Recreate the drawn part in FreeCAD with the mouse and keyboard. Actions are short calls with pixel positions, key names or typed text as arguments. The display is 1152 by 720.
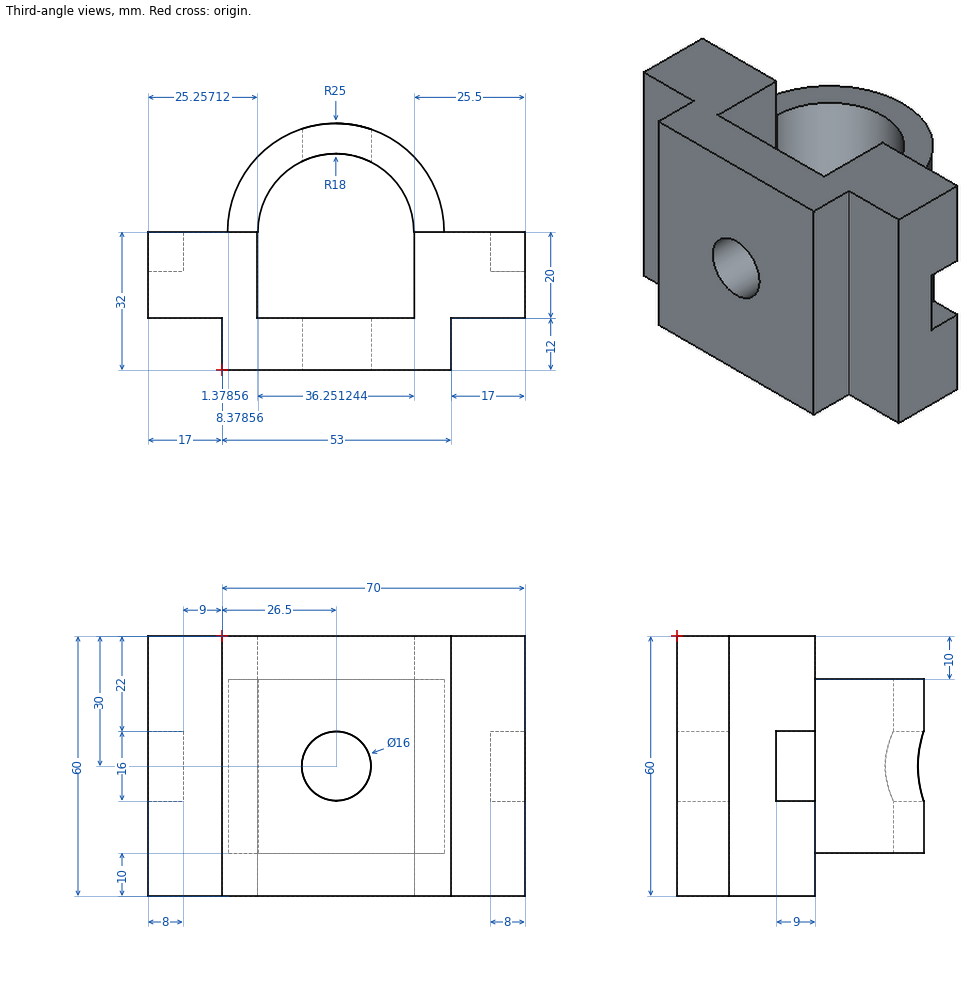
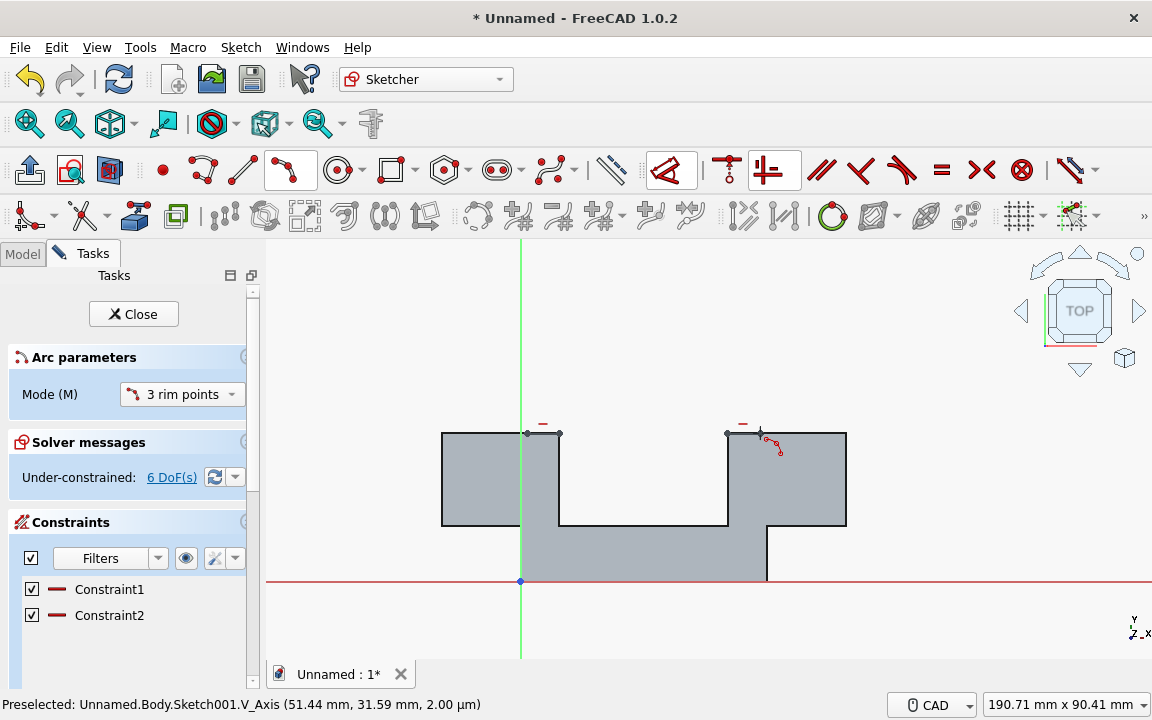
click(560, 434)
click(727, 434)
click(644, 349)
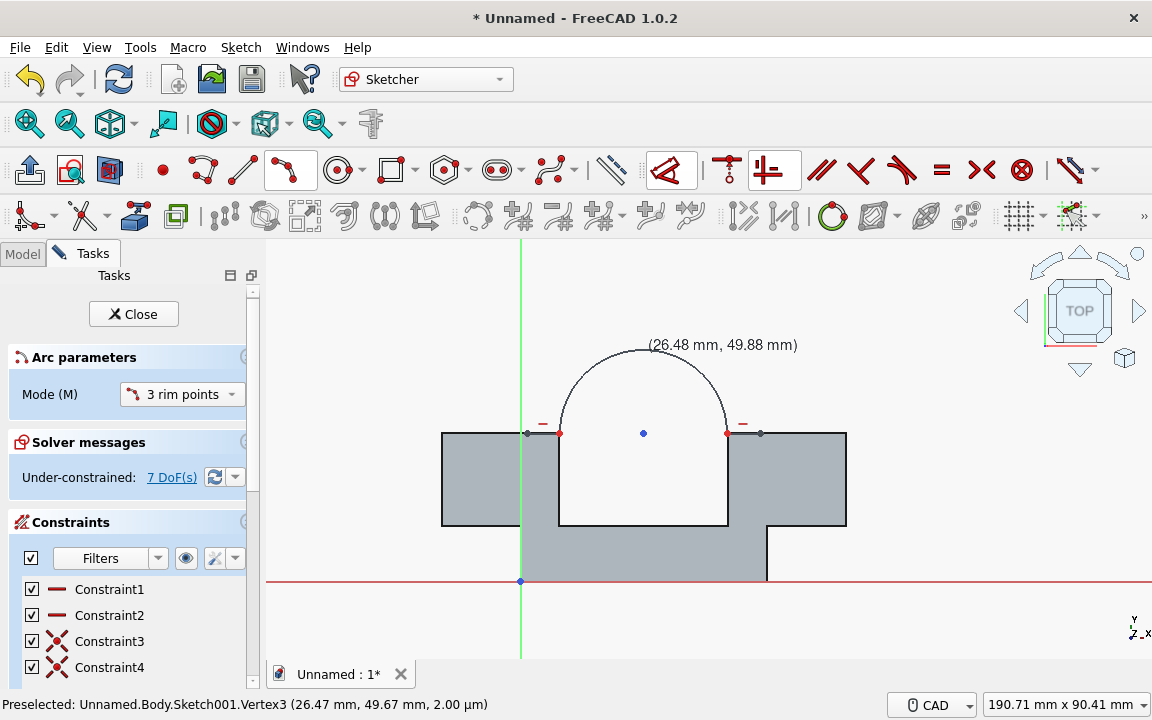
click(760, 434)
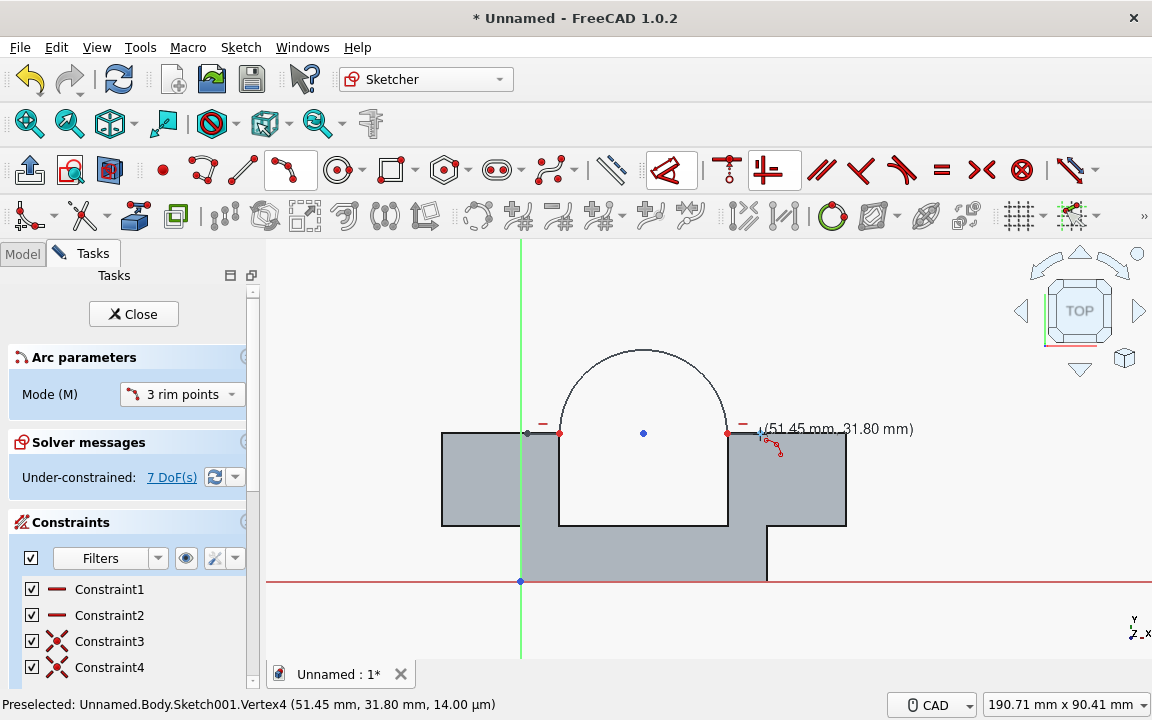
scroll(527, 433, up, 5)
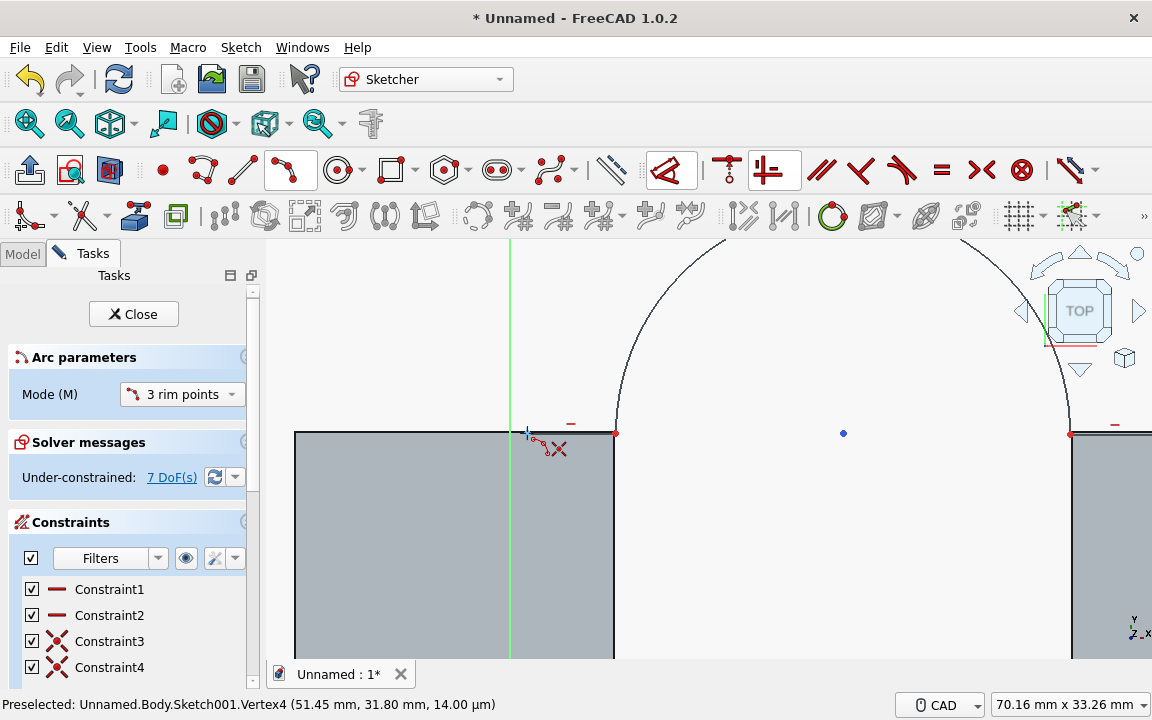
click(528, 434)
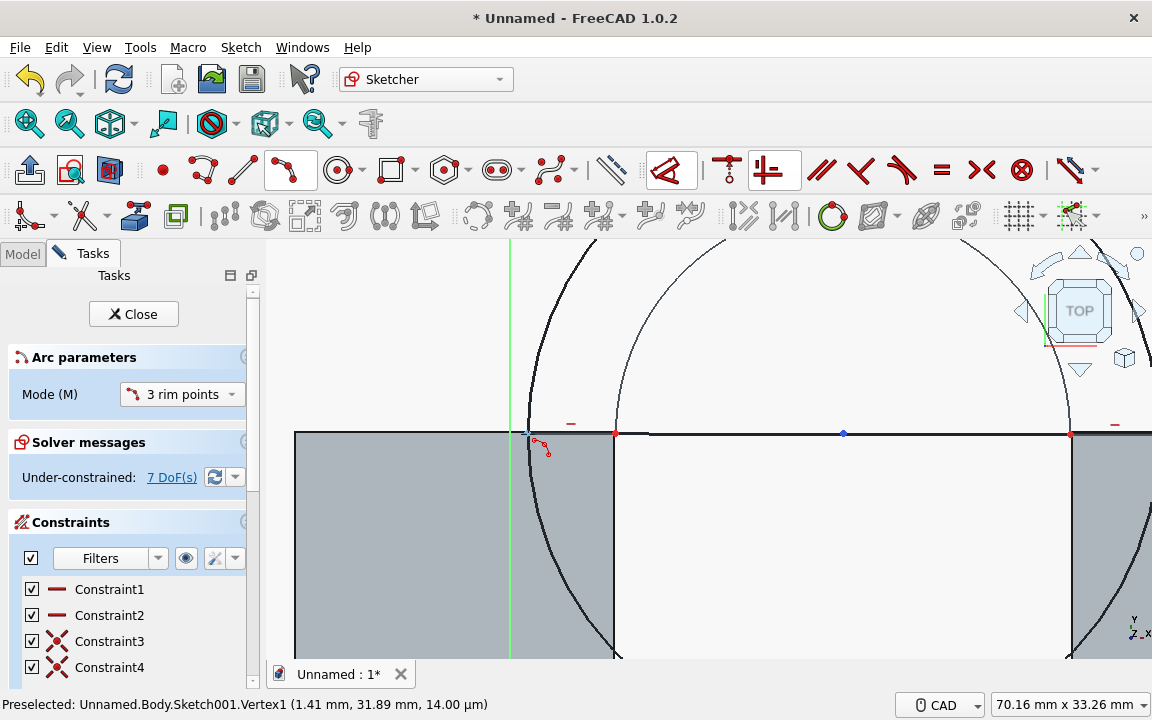
scroll(528, 433, down, 5)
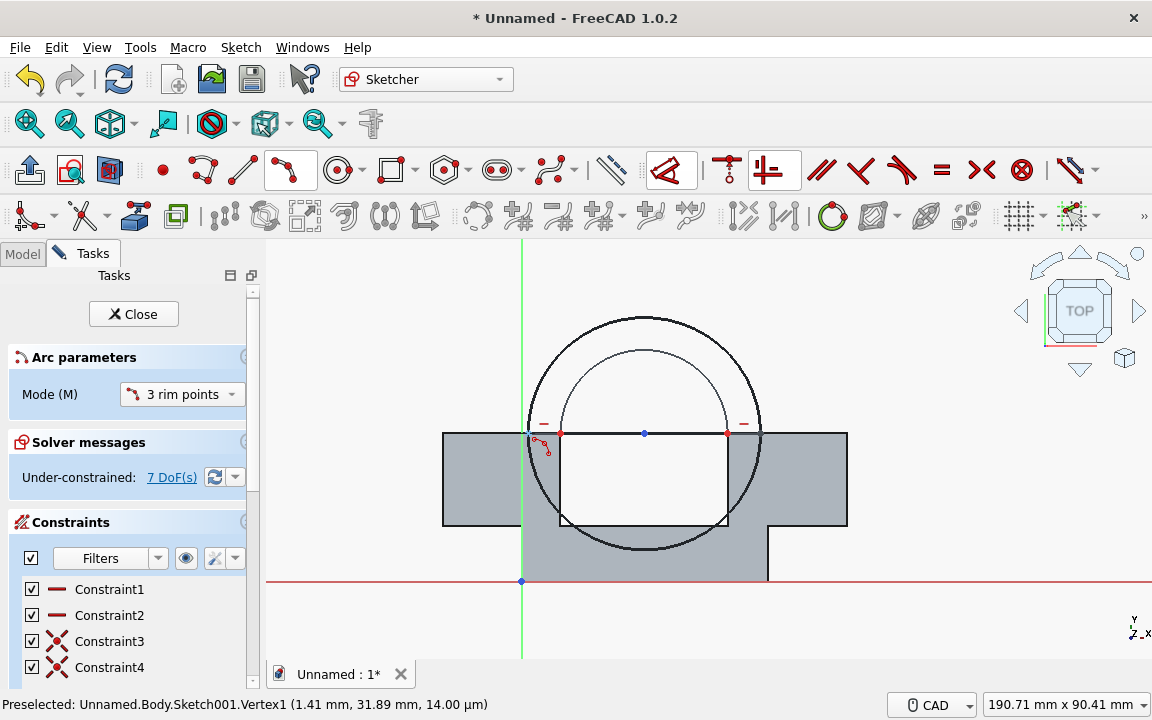
click(644, 317)
key(Escape)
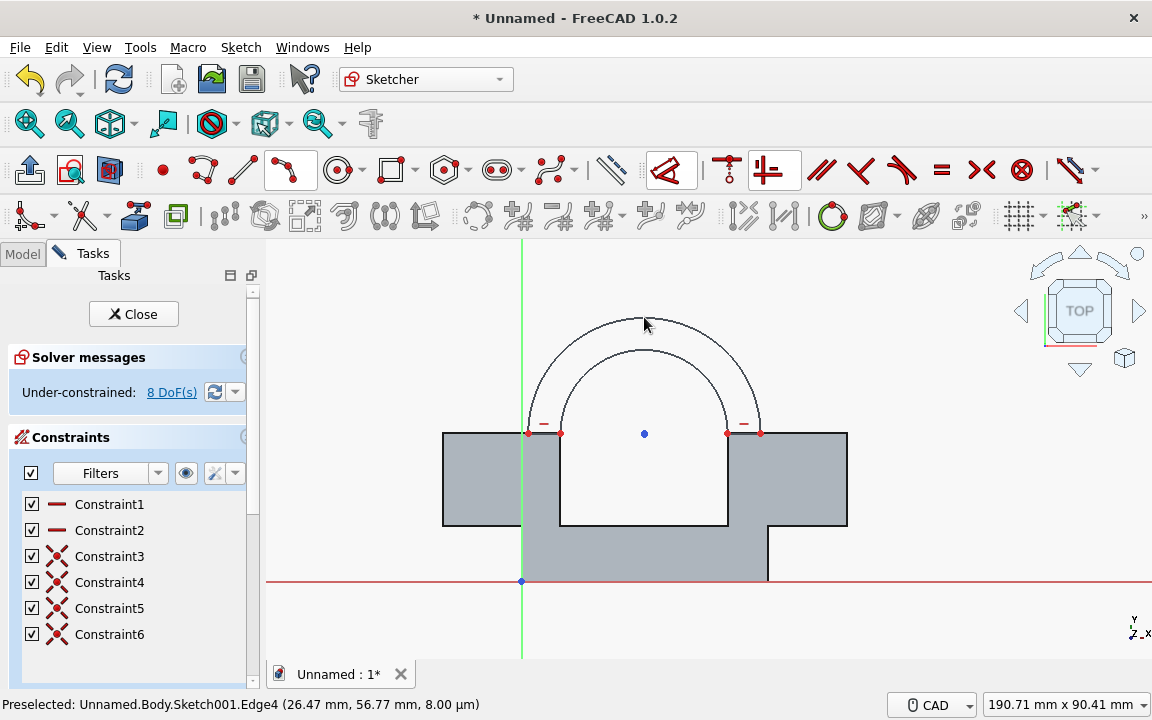
click(693, 366)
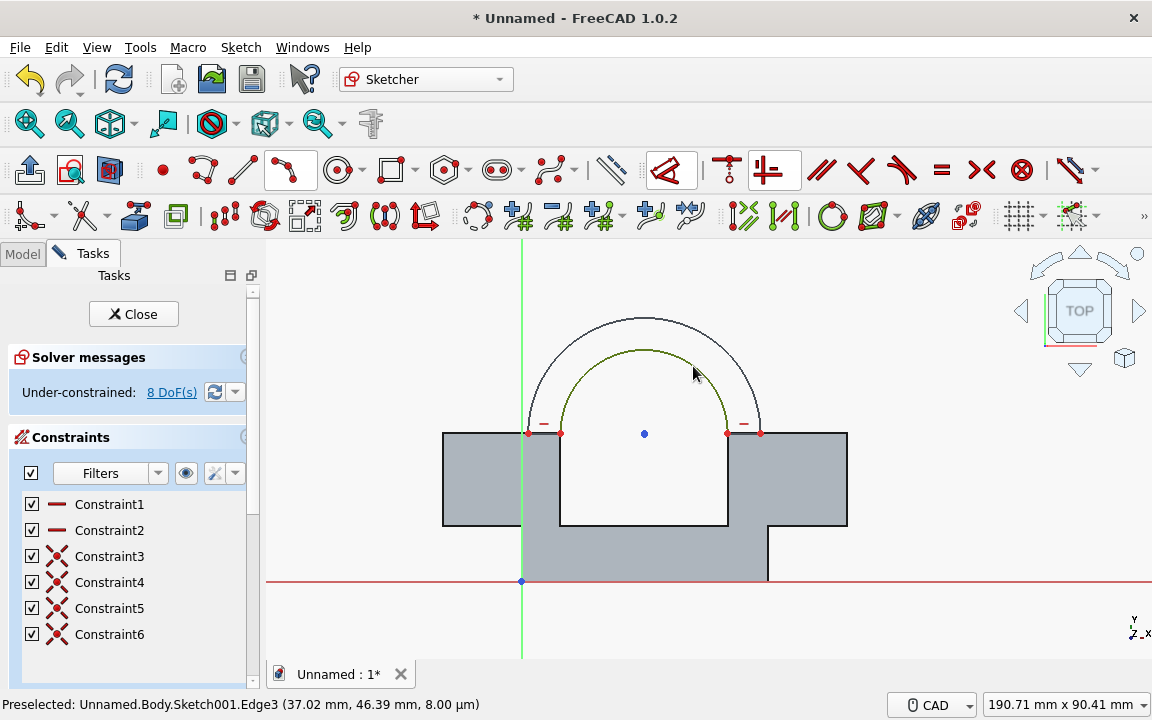
click(713, 340)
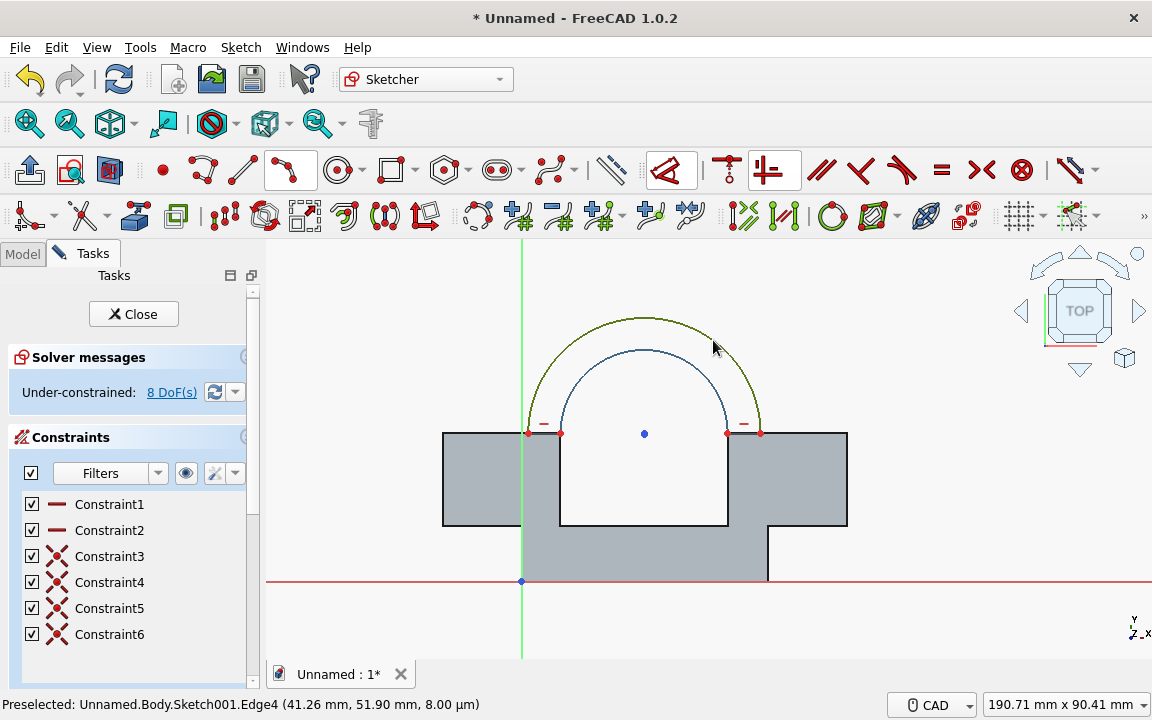
key(c)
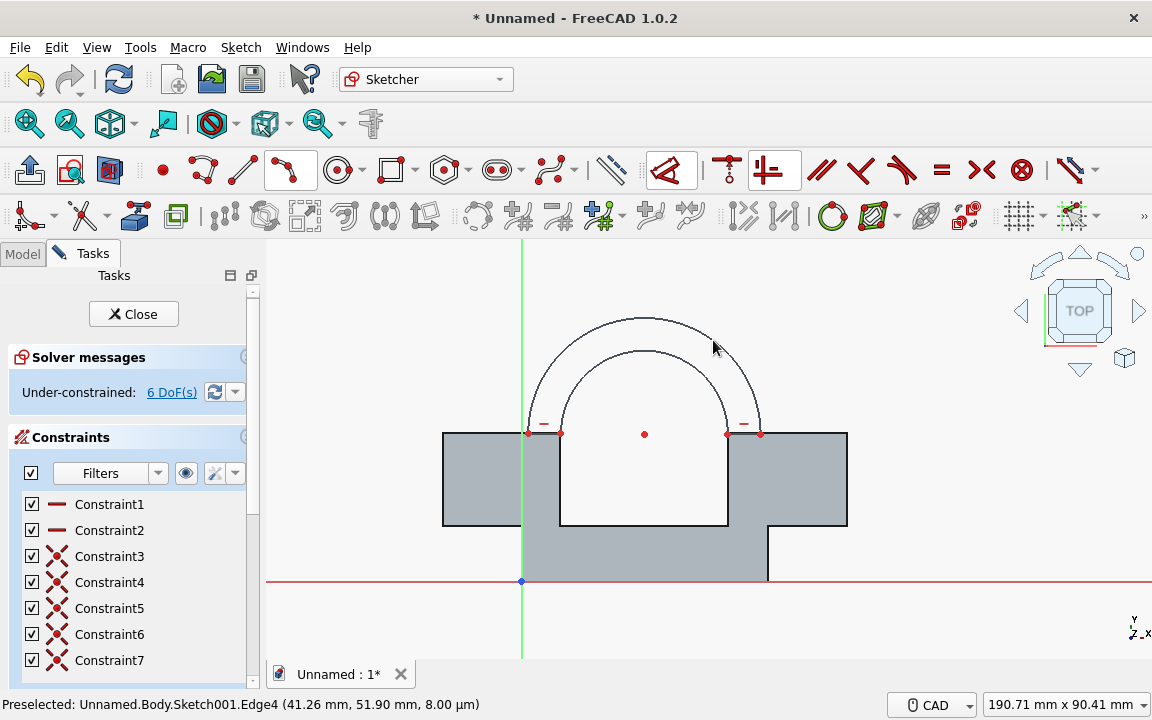
click(694, 367)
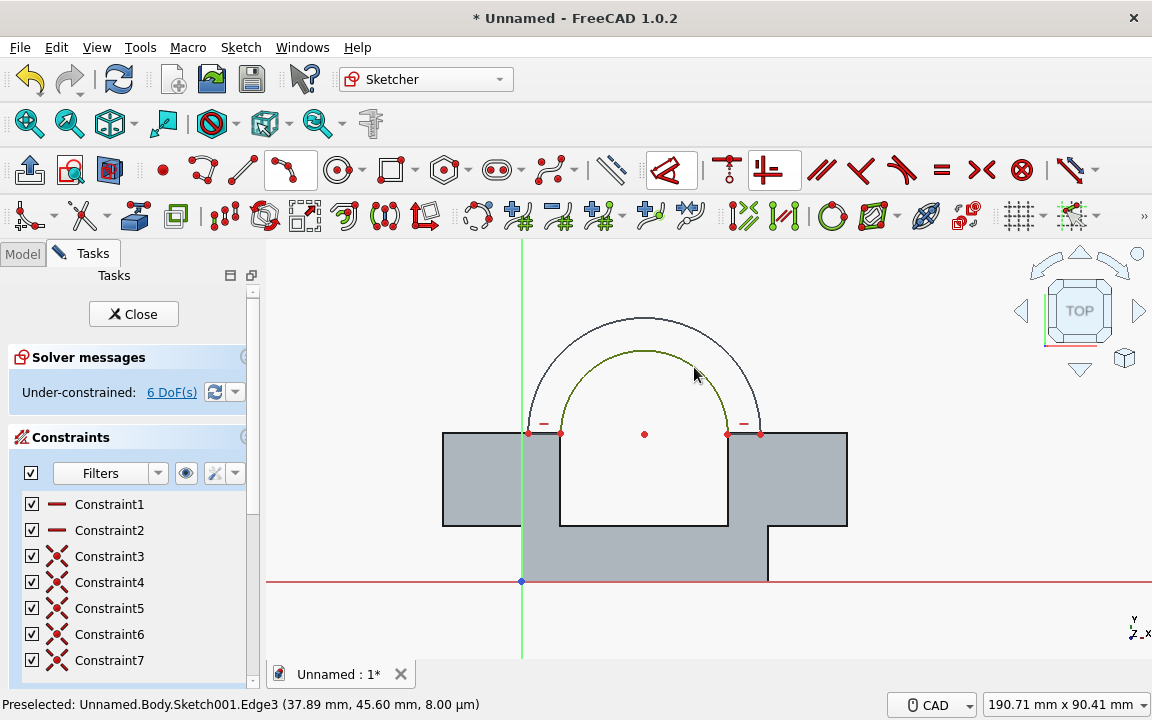
key(k)
key(r)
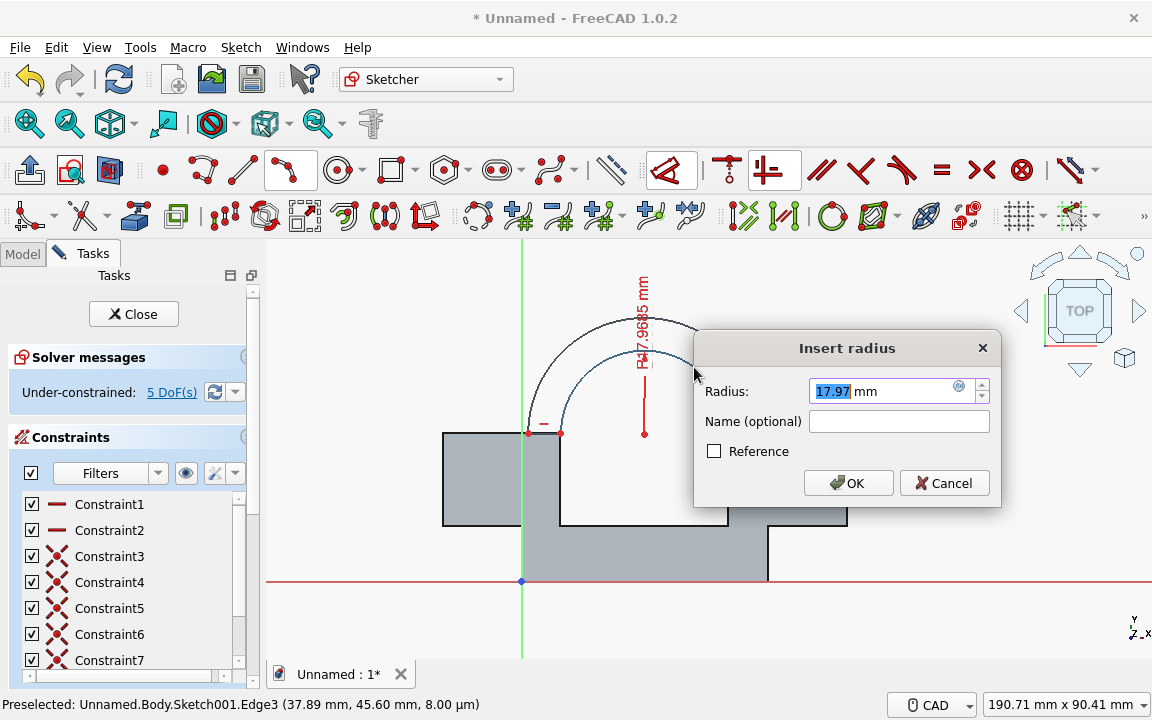
text(18)
key(Return)